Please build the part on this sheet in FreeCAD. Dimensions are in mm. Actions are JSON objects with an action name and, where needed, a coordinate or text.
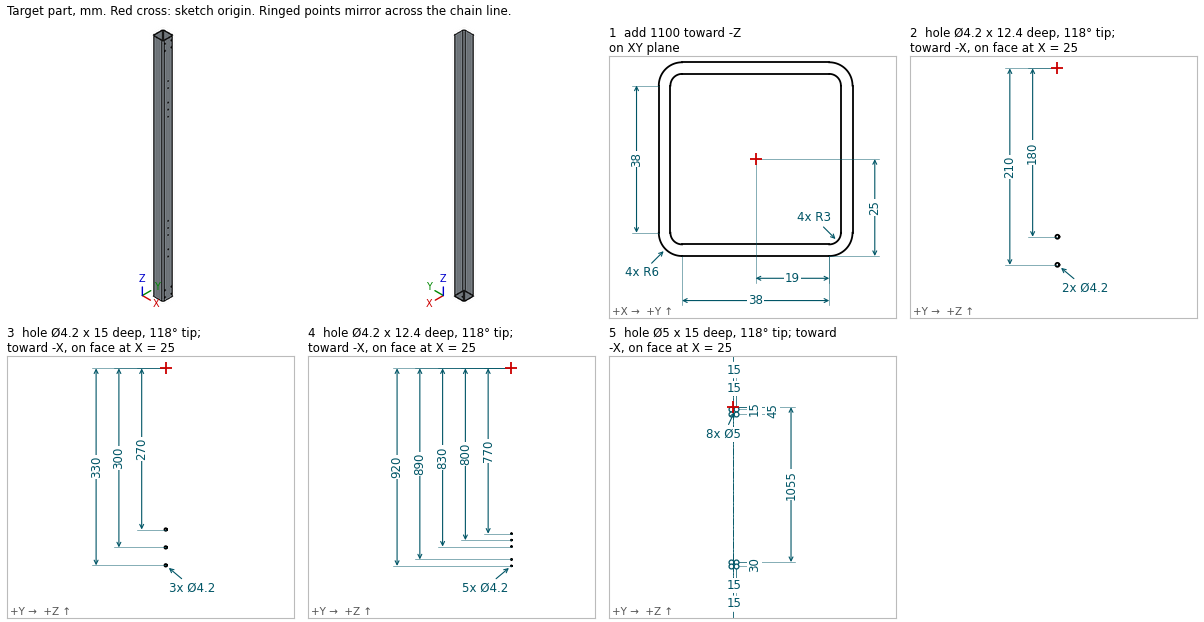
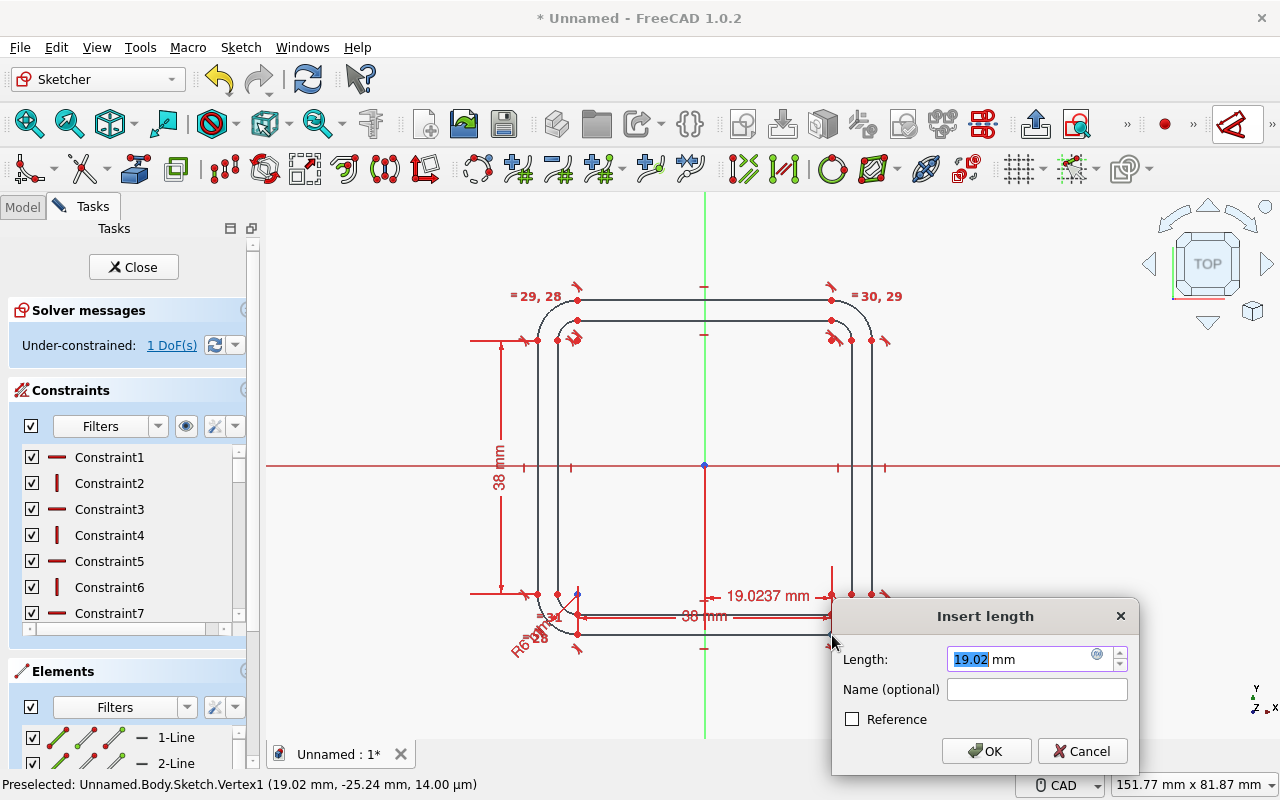
{"action": "type", "text": "19"}
{"action": "key", "text": "Return"}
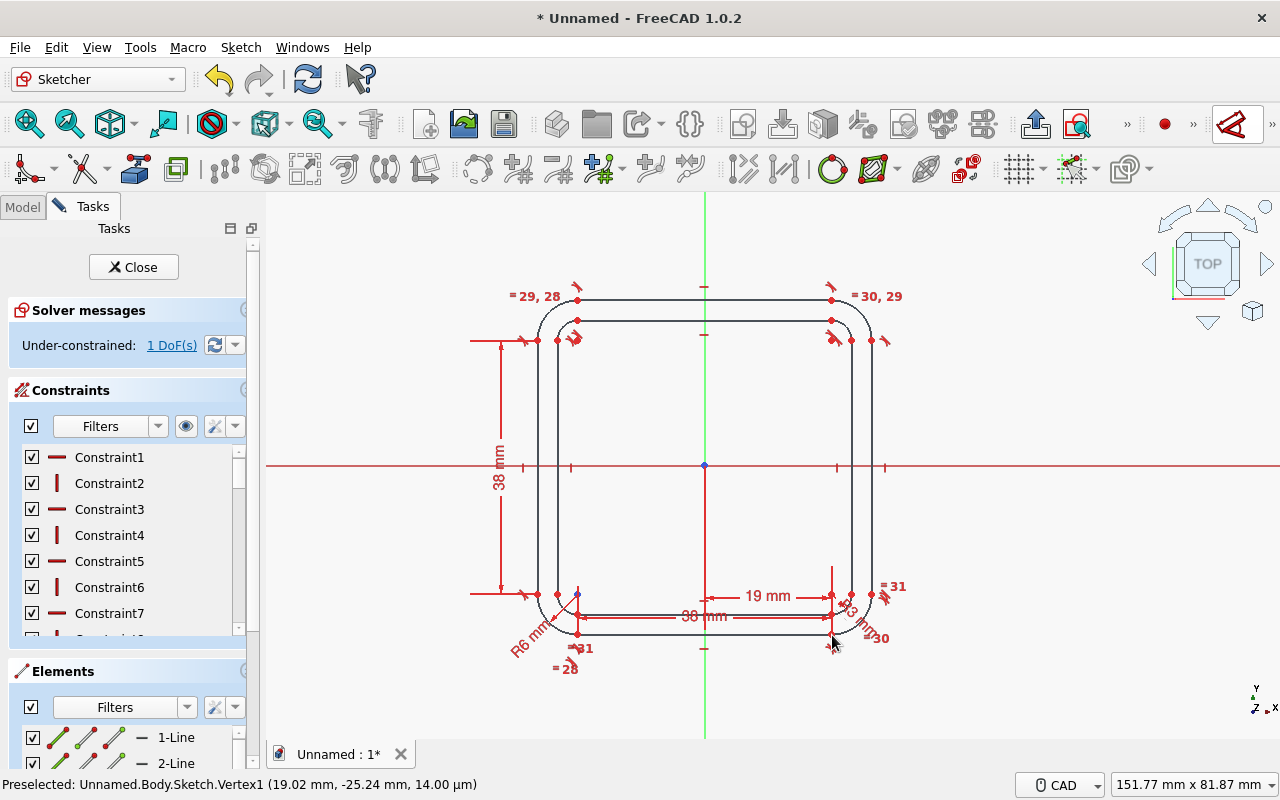
{"action": "left_click", "coordinate": [832, 635]}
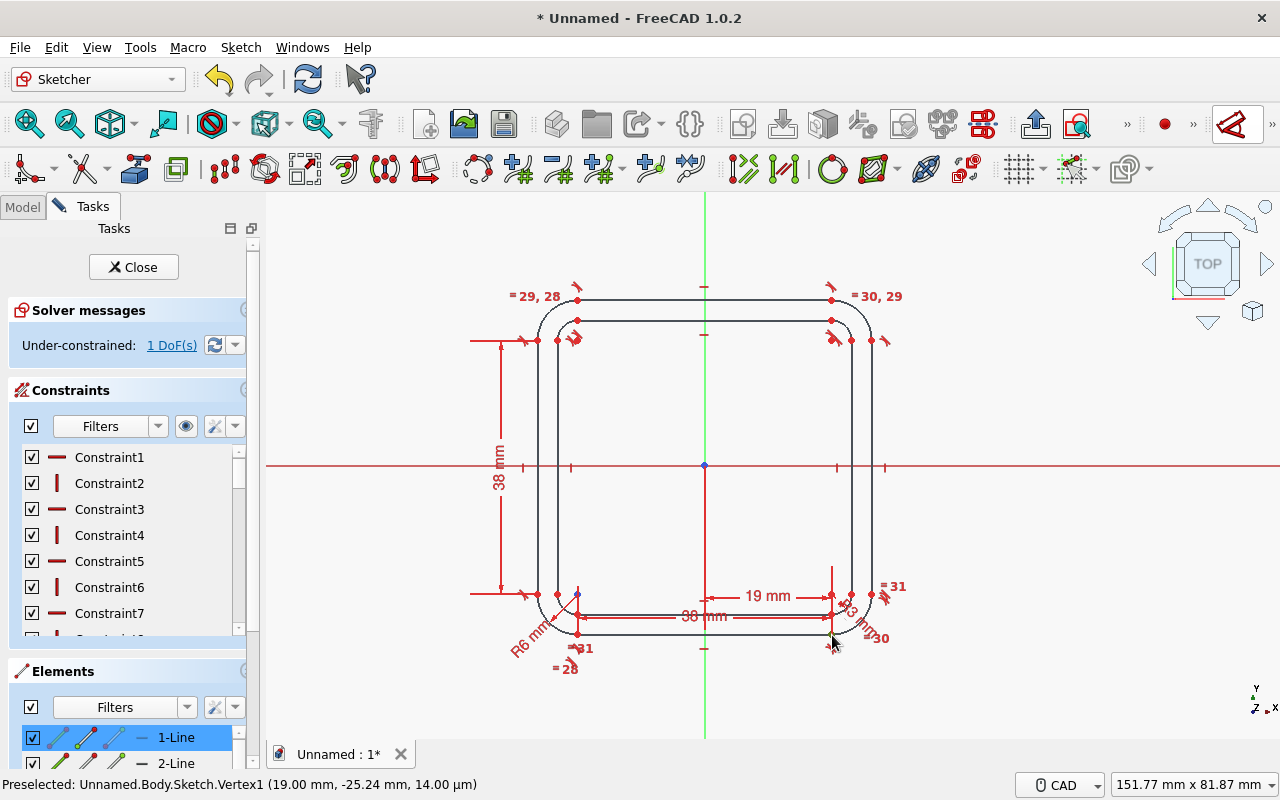
{"action": "left_click", "coordinate": [1258, 124]}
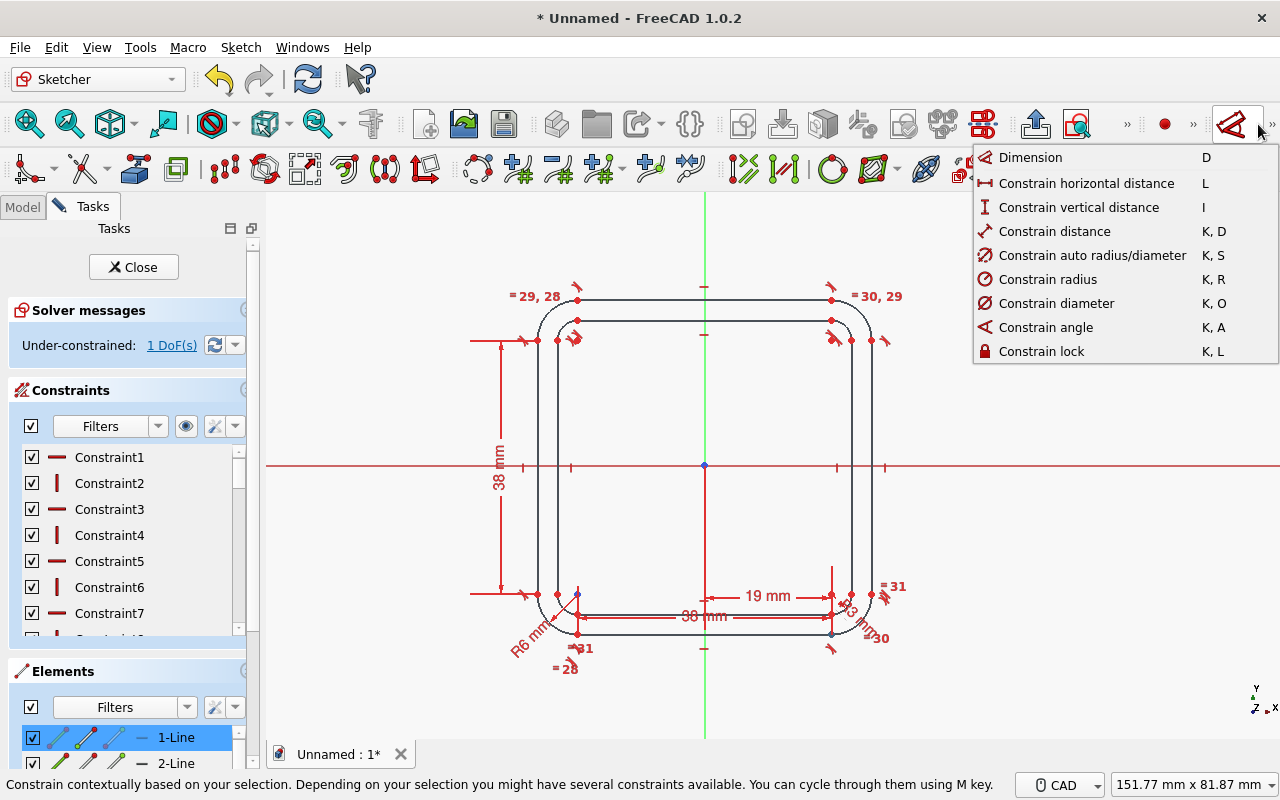
{"action": "left_click", "coordinate": [1126, 207]}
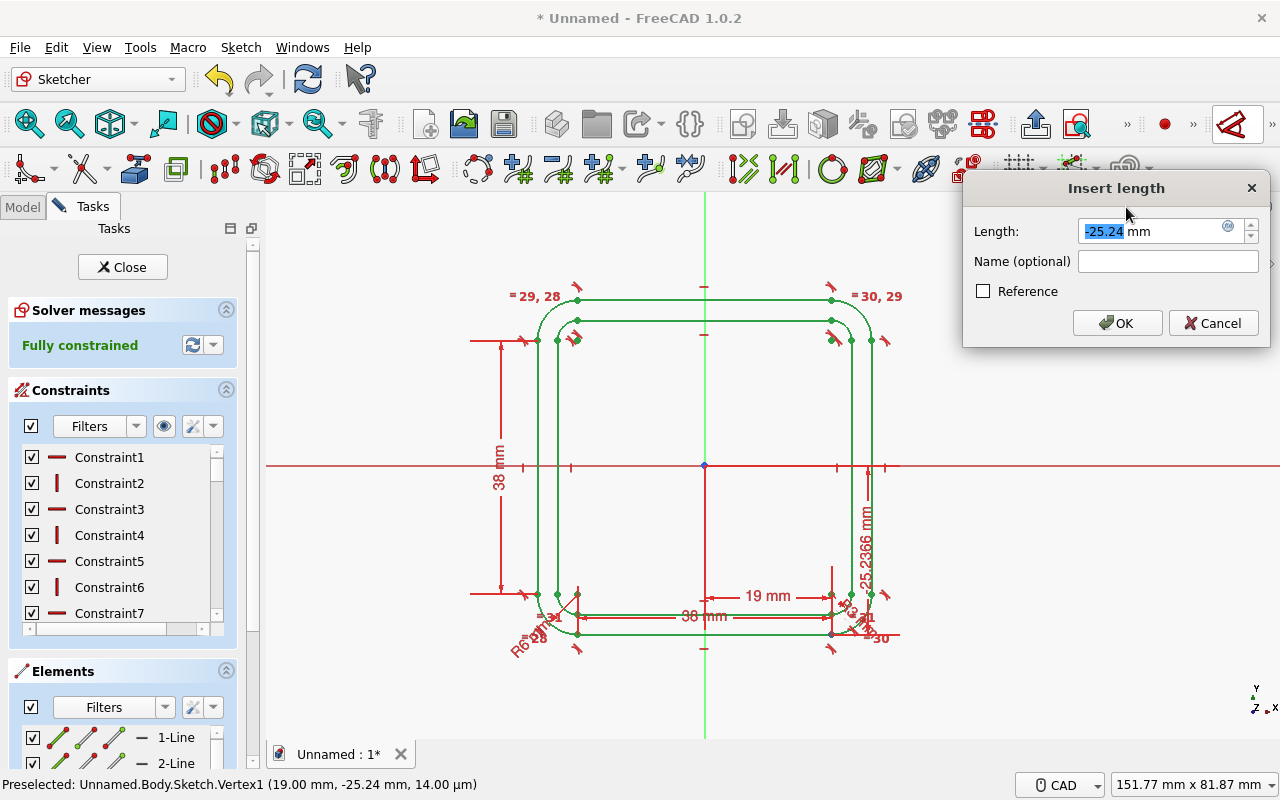
{"action": "type", "text": "-25"}
{"action": "key", "text": "Return"}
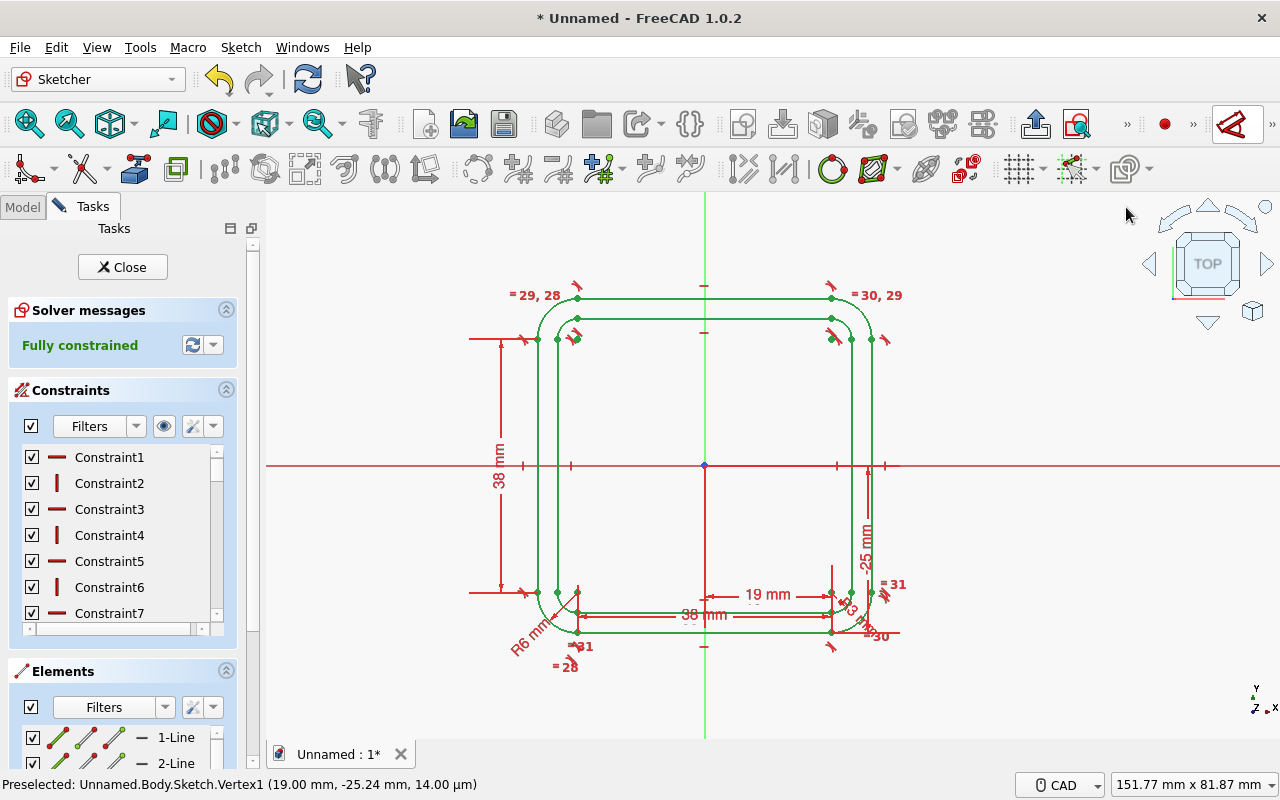
{"action": "left_click", "coordinate": [123, 267]}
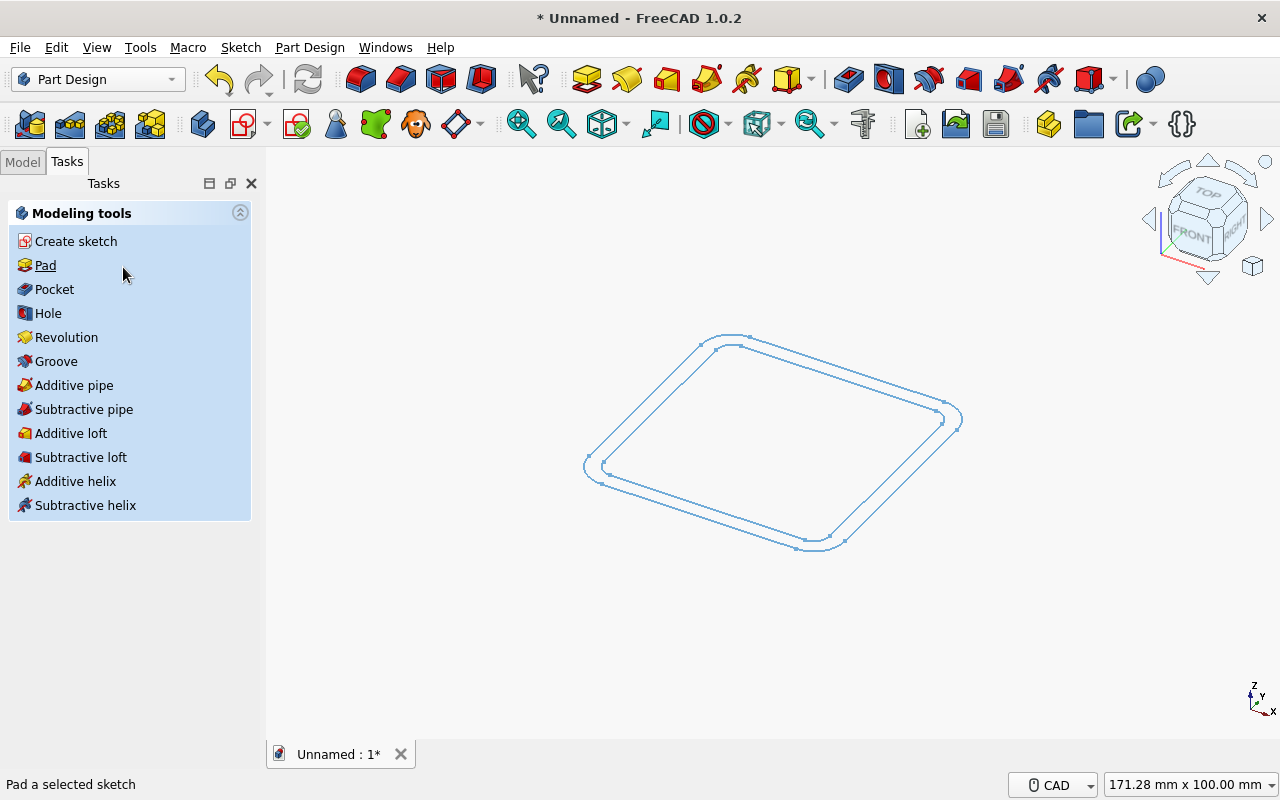
{"action": "left_click", "coordinate": [588, 80]}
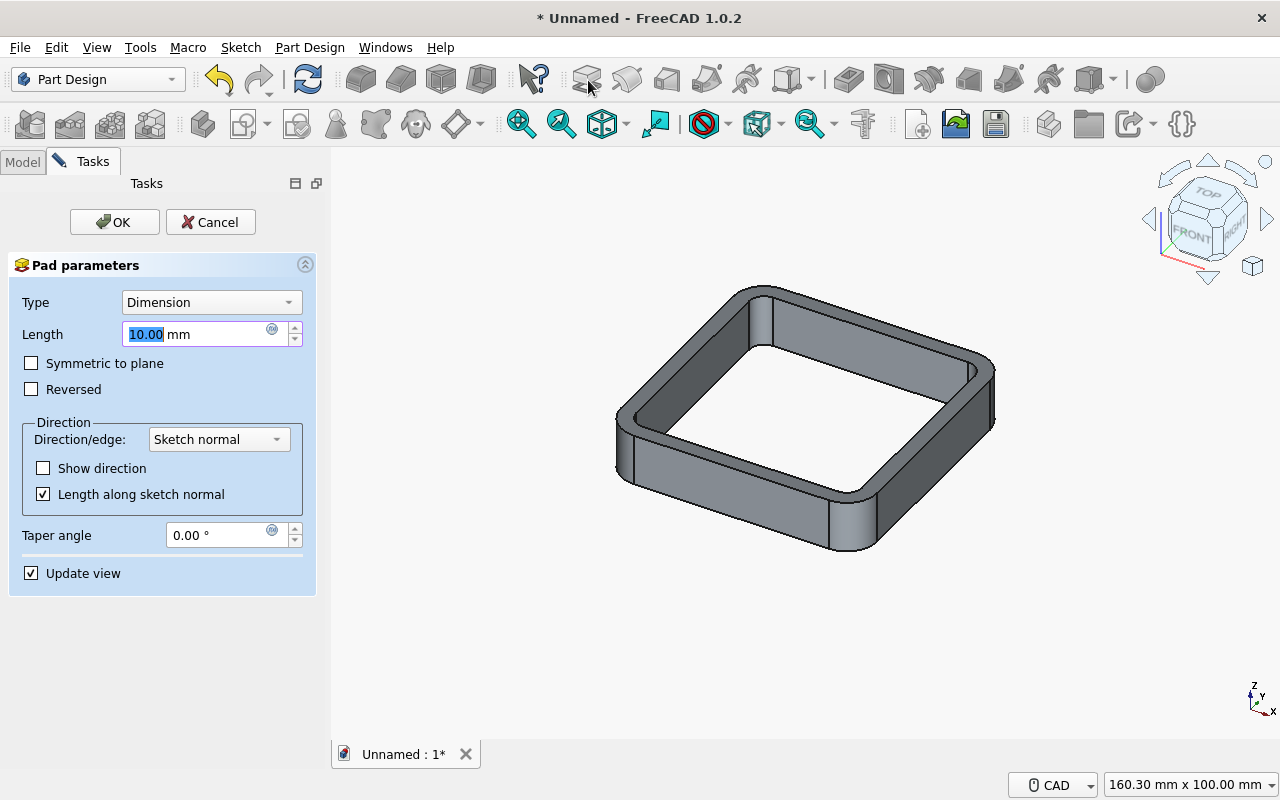
{"action": "type", "text": "1100"}
{"action": "key", "text": "Tab"}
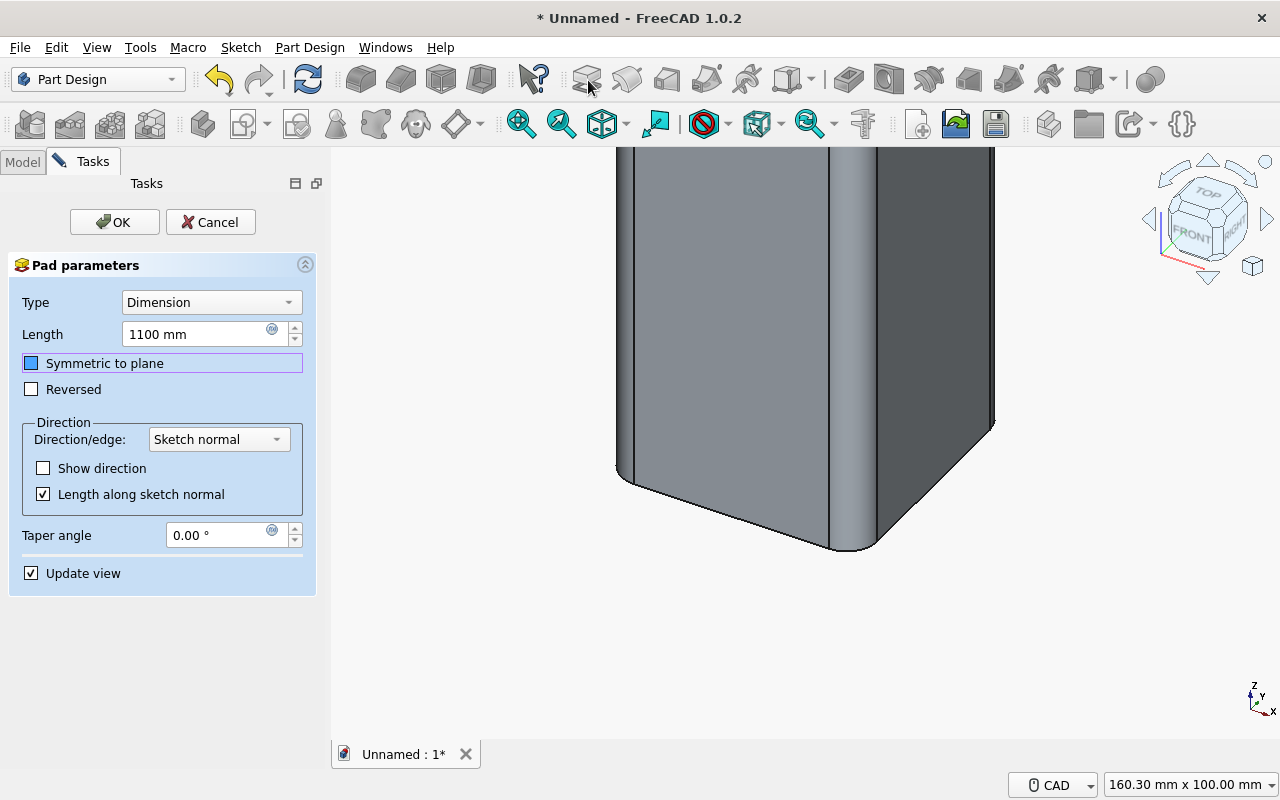
{"action": "left_click", "coordinate": [30, 389]}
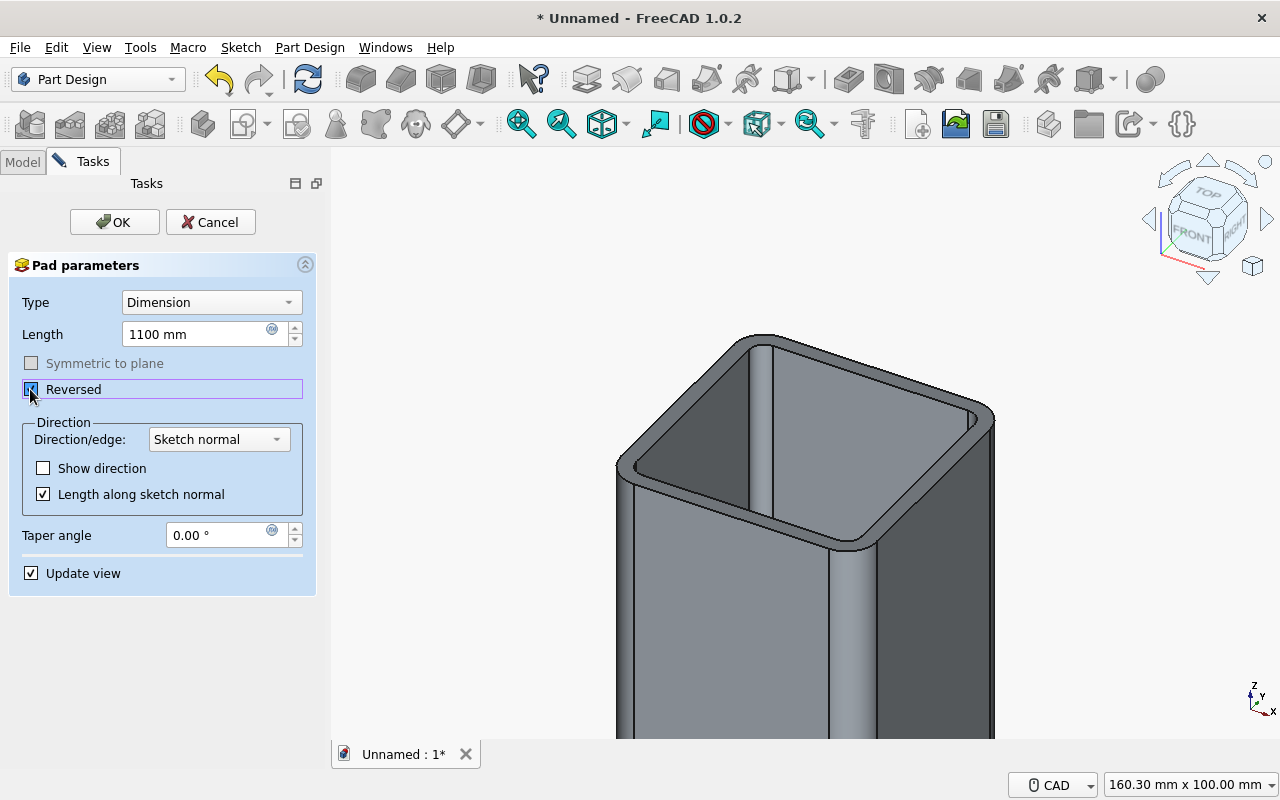
{"action": "left_click", "coordinate": [115, 222]}